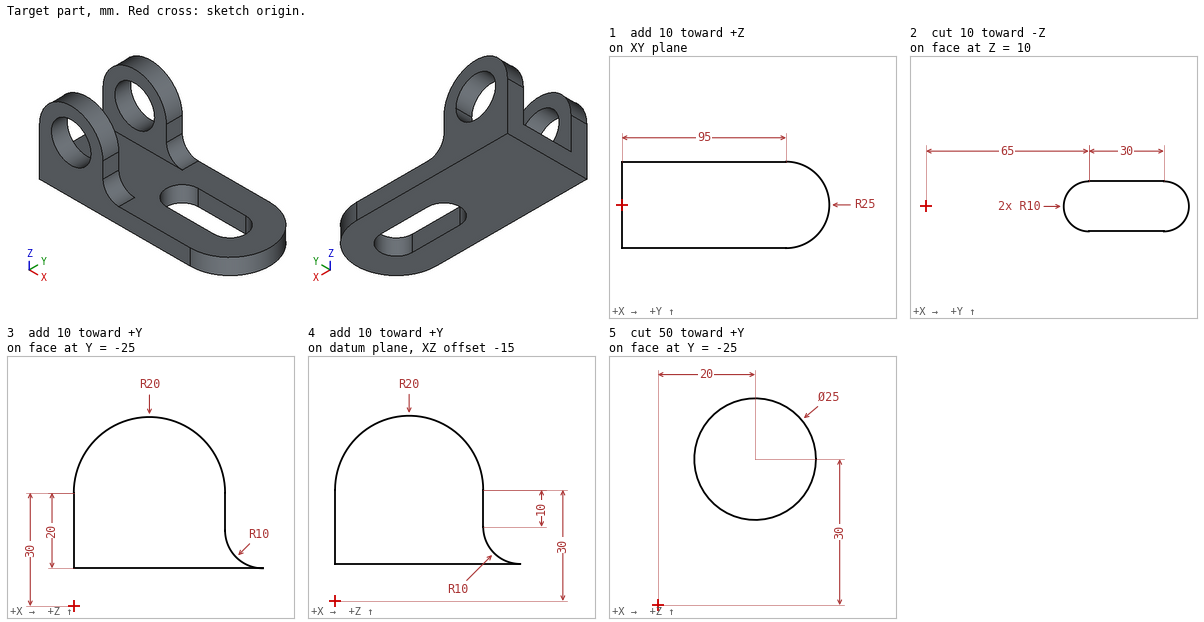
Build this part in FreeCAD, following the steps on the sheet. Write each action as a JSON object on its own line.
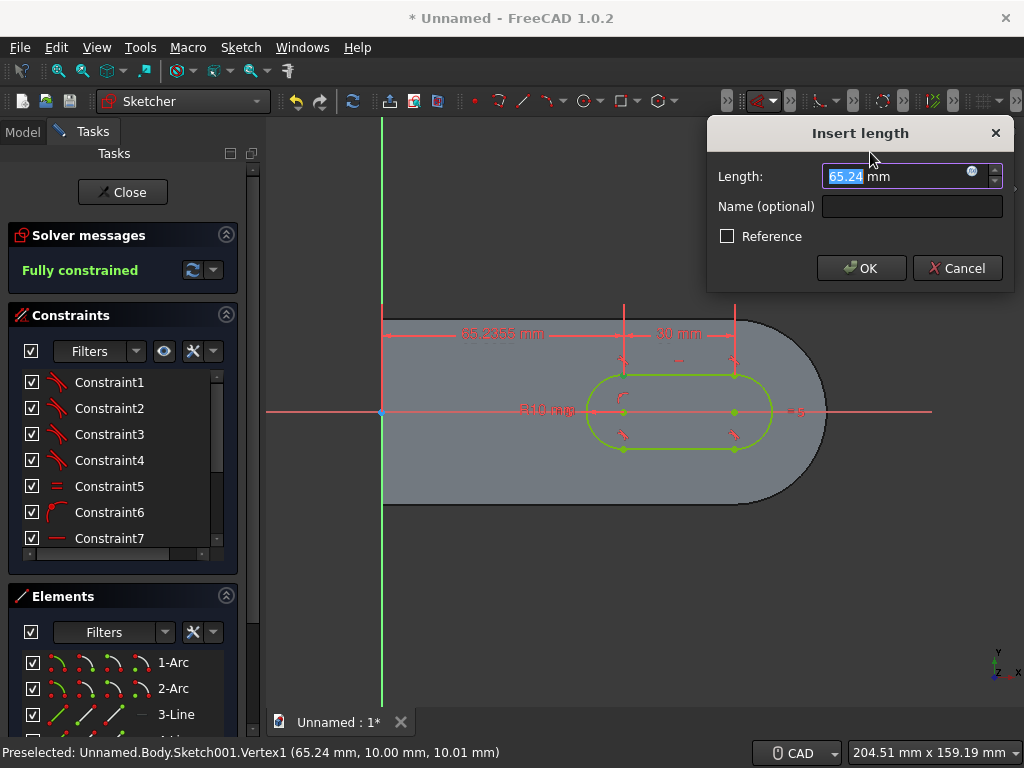
{"action": "type", "text": "65"}
{"action": "key", "text": "Return"}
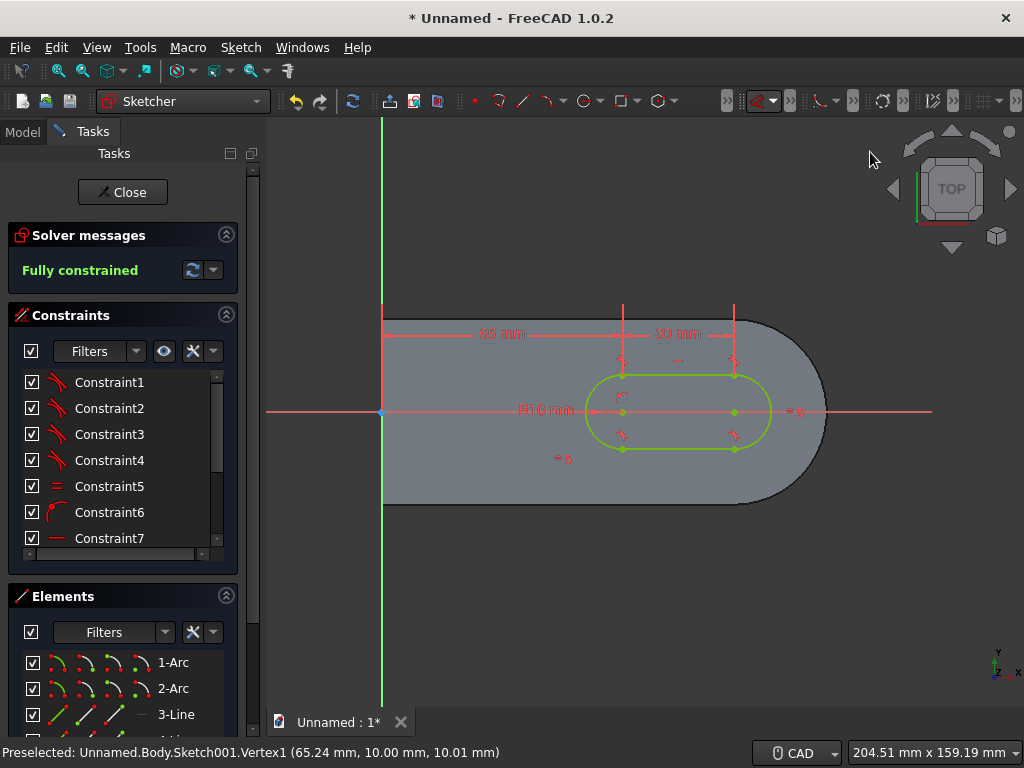
{"action": "left_click", "coordinate": [123, 192]}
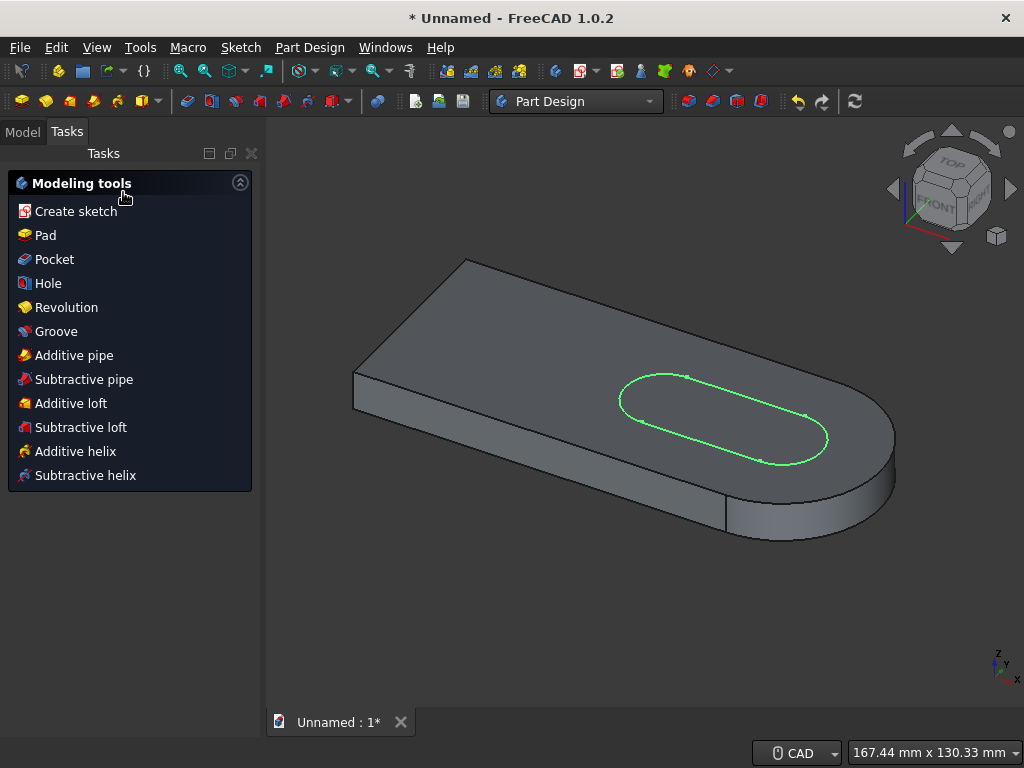
{"action": "left_click", "coordinate": [188, 102]}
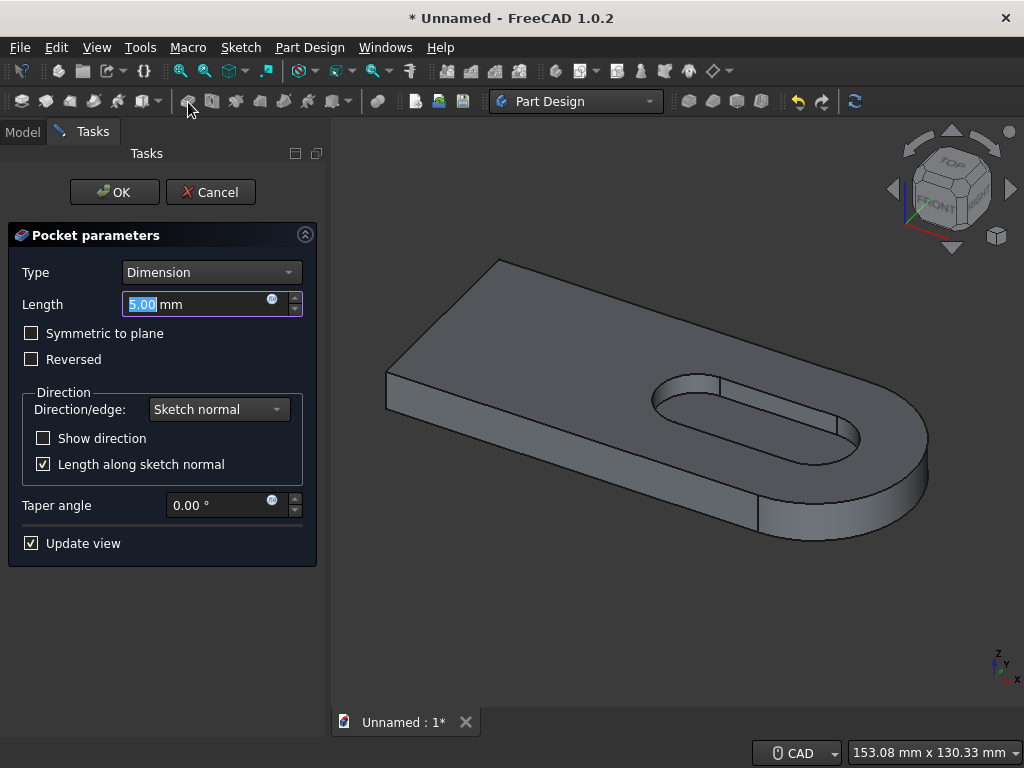
{"action": "type", "text": "10"}
{"action": "key", "text": "Tab"}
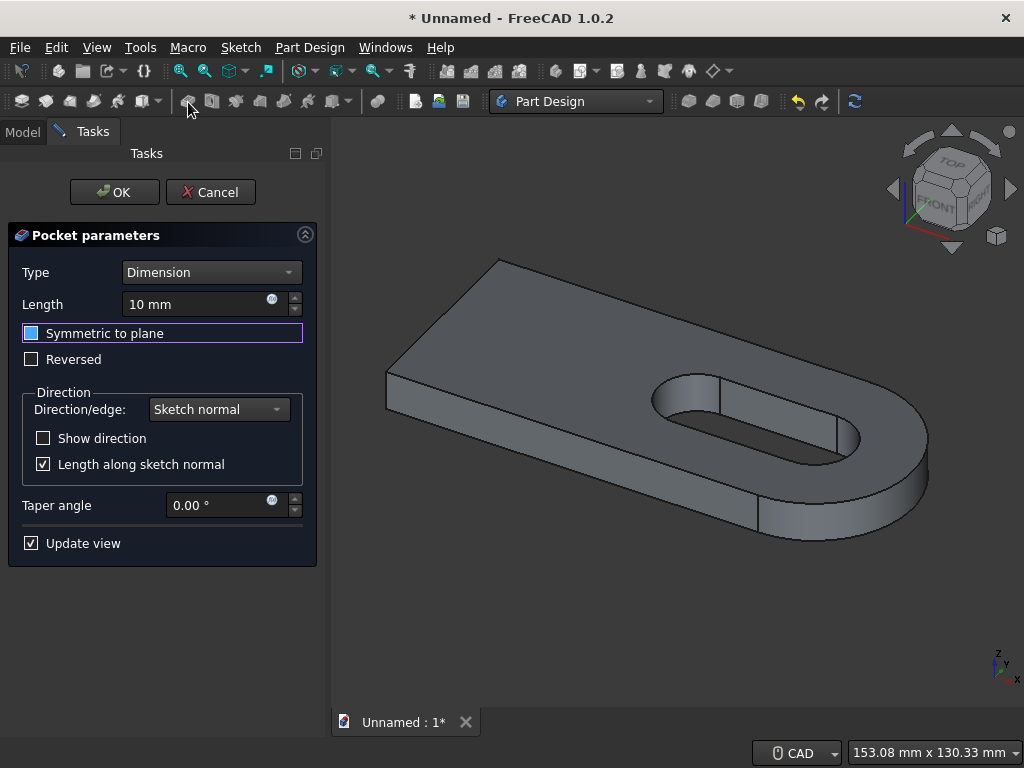
{"action": "left_click", "coordinate": [115, 192]}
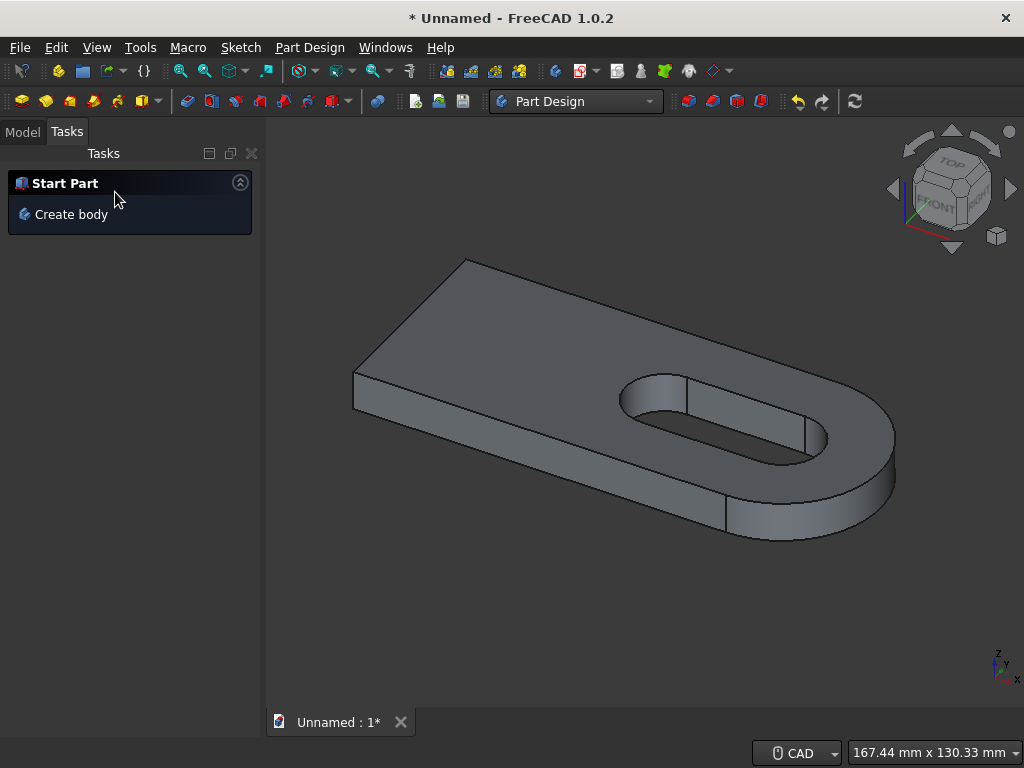
{"action": "left_click", "coordinate": [699, 504]}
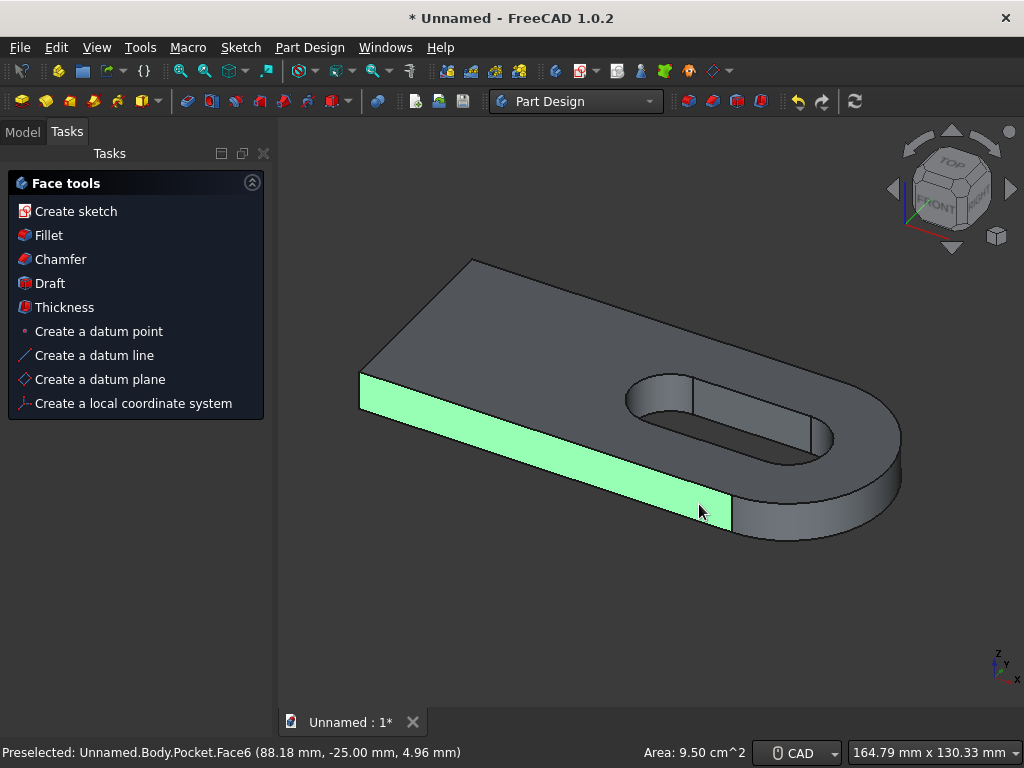
{"action": "left_click", "coordinate": [580, 72]}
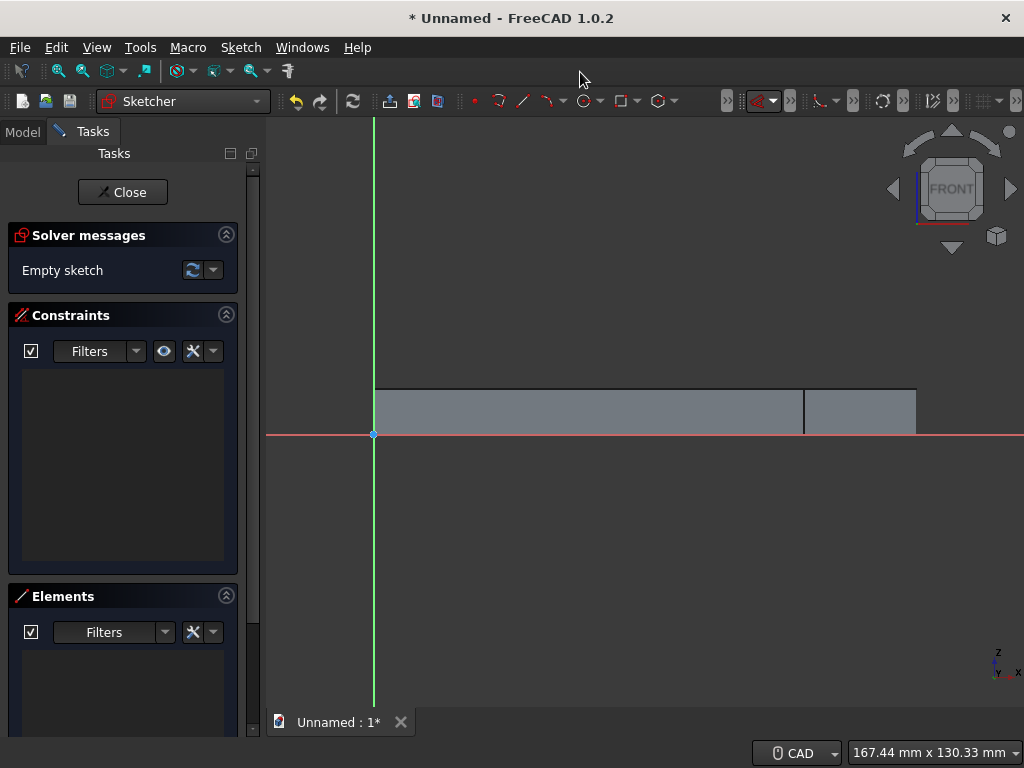
{"action": "scroll", "coordinate": [377, 211], "scroll_direction": "up", "scroll_amount": 3}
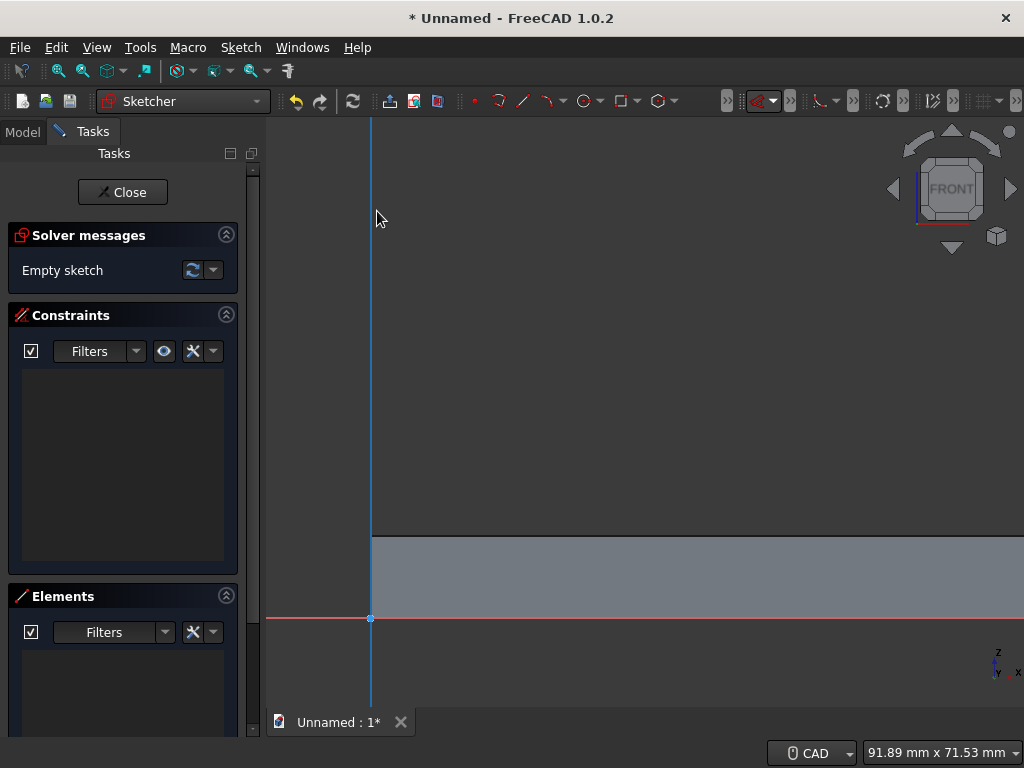
{"action": "left_click", "coordinate": [500, 102]}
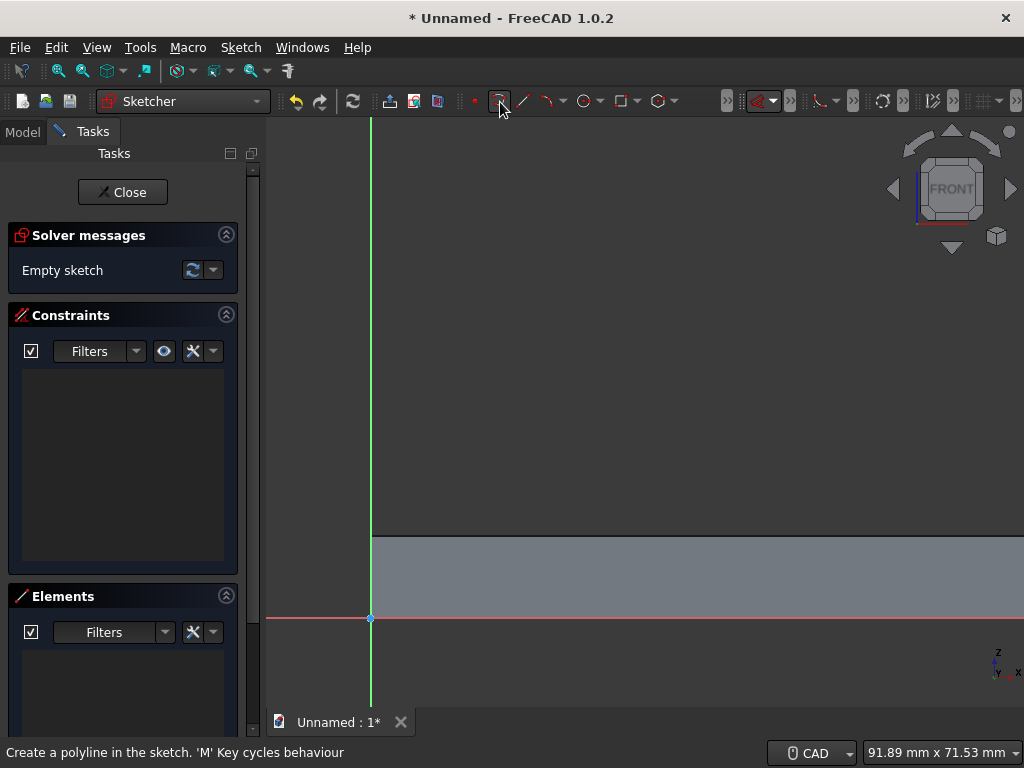
{"action": "left_click", "coordinate": [371, 371]}
{"action": "left_click", "coordinate": [380, 536]}
{"action": "left_click", "coordinate": [783, 536]}
{"action": "right_click", "coordinate": [783, 536]}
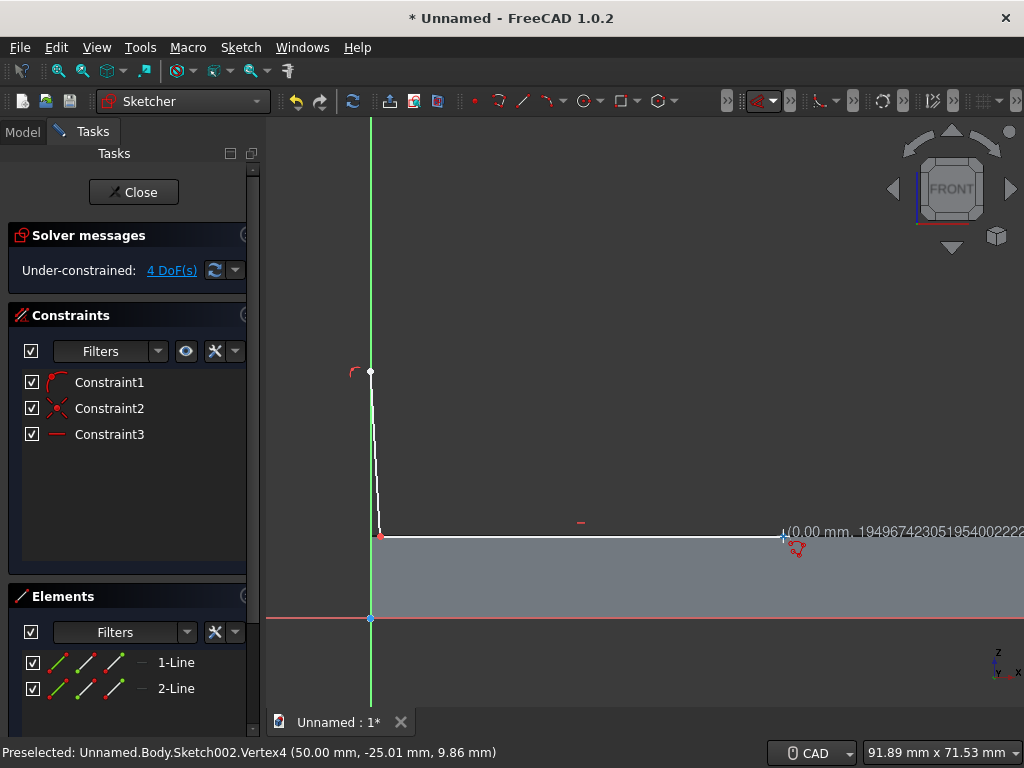
{"action": "left_click", "coordinate": [524, 102]}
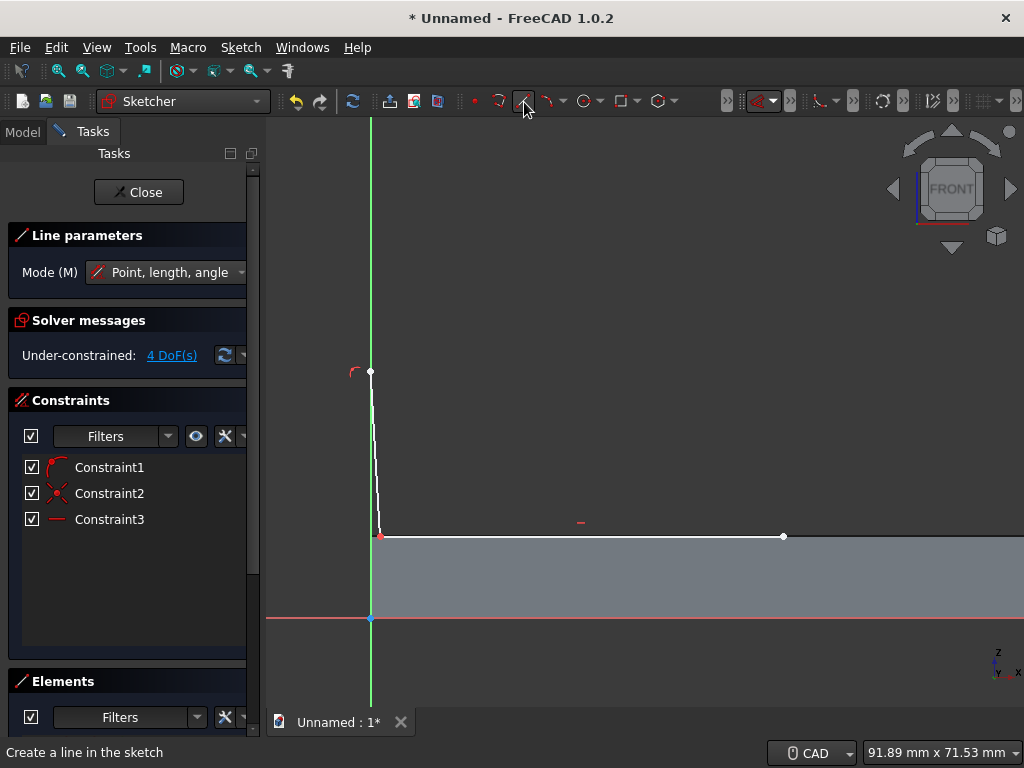
{"action": "left_click", "coordinate": [700, 453]}
{"action": "left_click", "coordinate": [700, 371]}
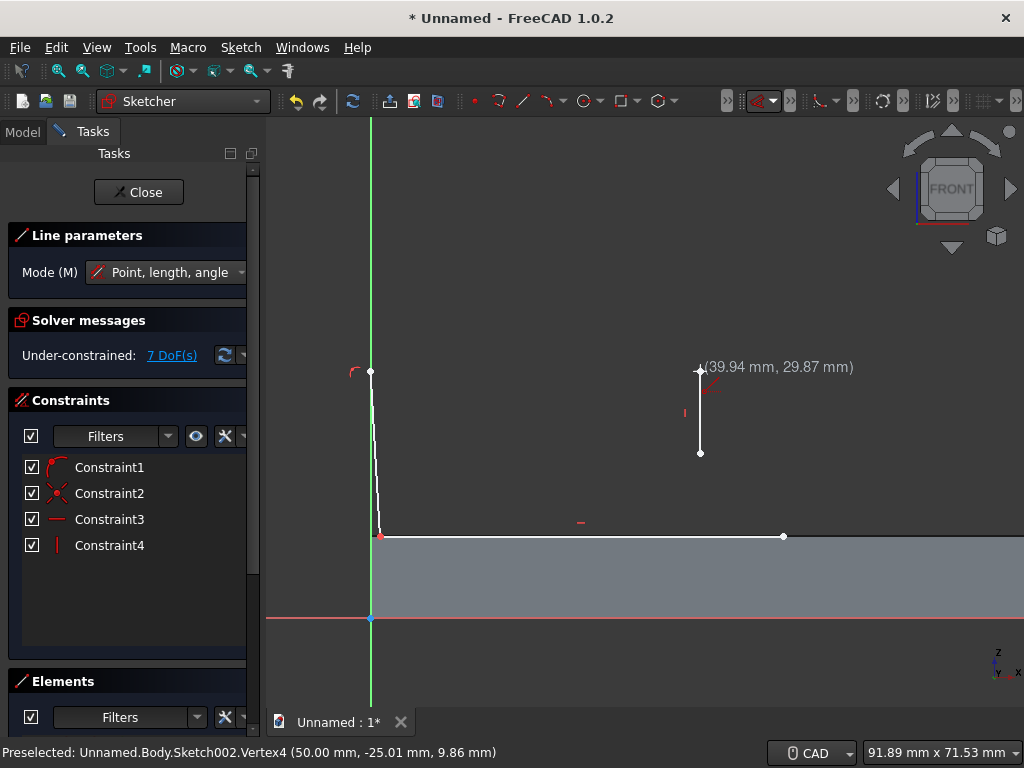
{"action": "left_click", "coordinate": [548, 102]}